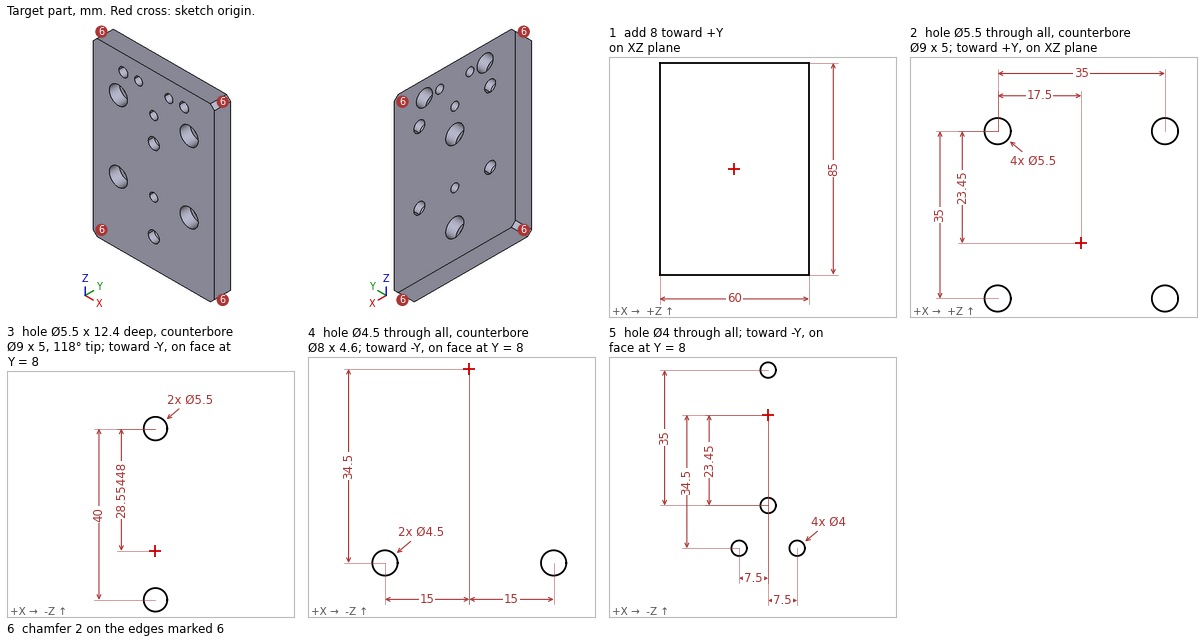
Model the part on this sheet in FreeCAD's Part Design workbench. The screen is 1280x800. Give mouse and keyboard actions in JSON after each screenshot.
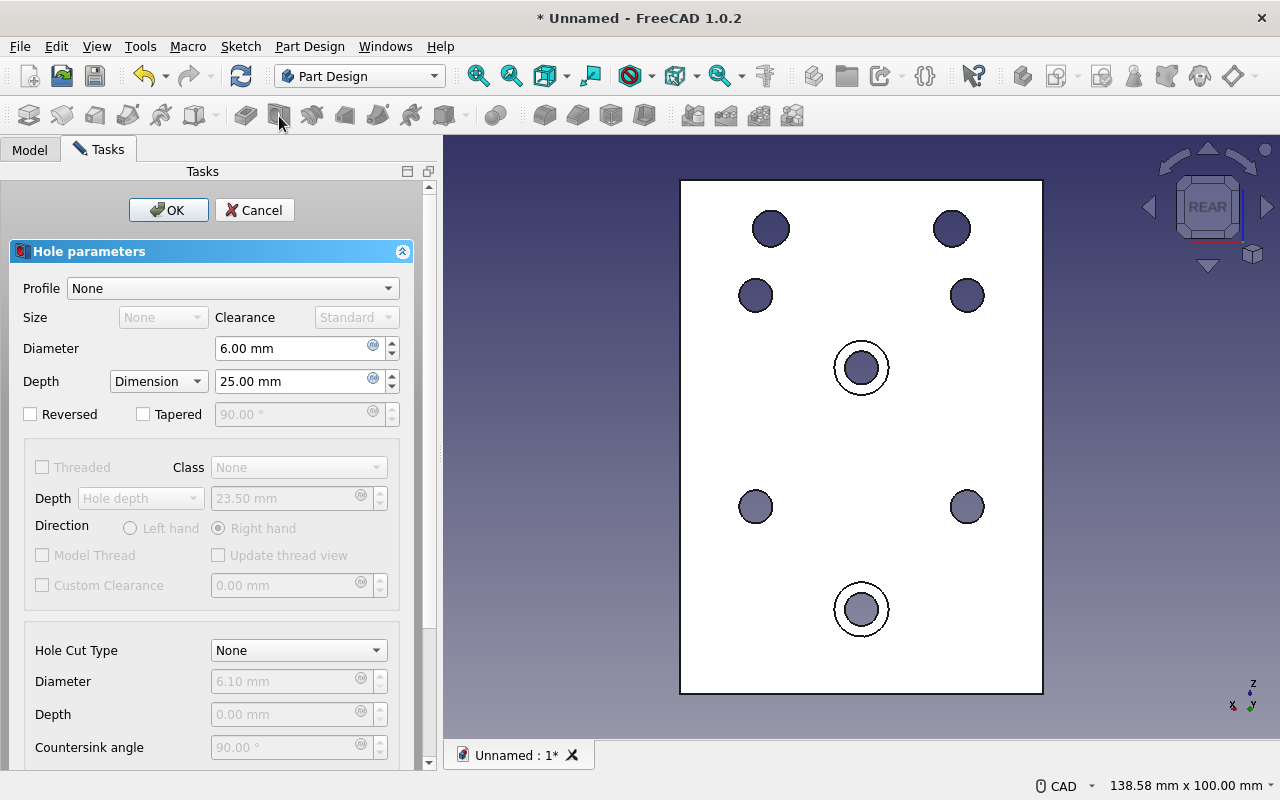
{"action": "triple_click", "coordinate": [300, 348]}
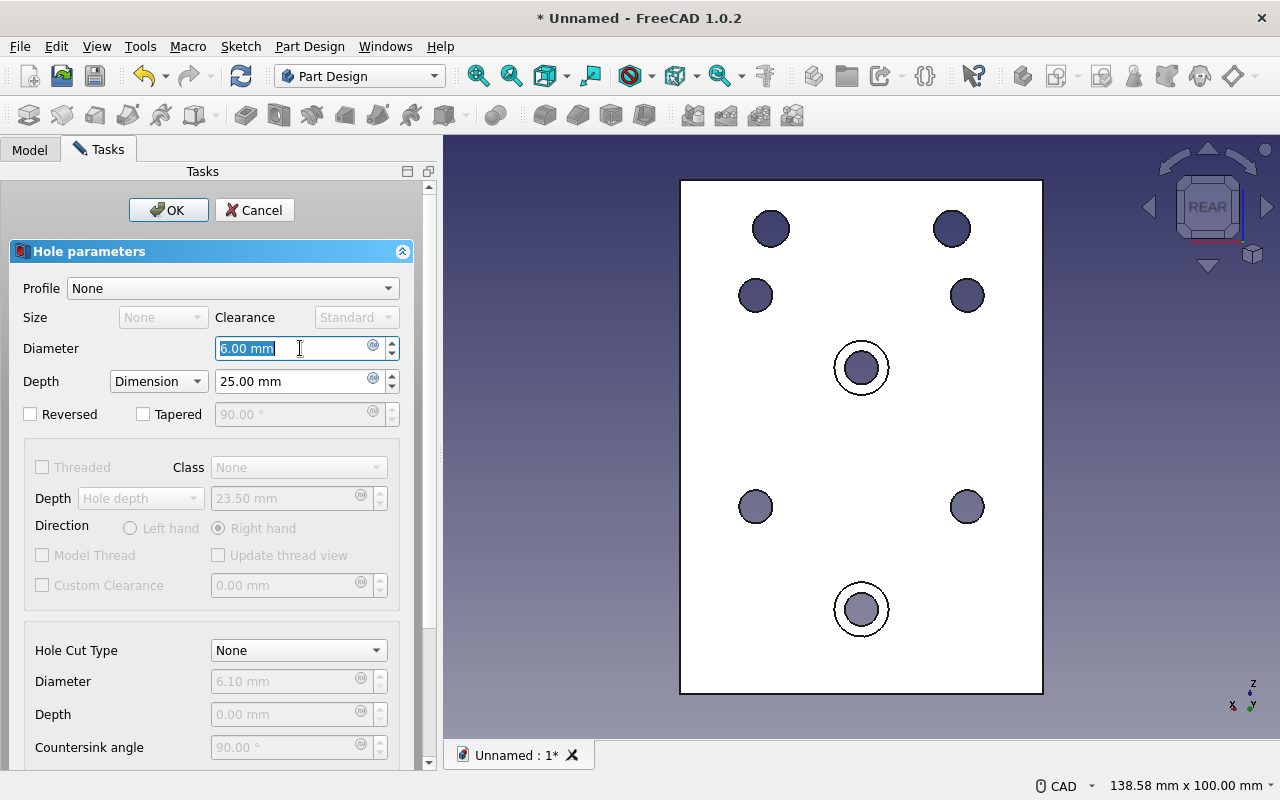
{"action": "type", "text": "4.5"}
{"action": "key", "text": "Tab"}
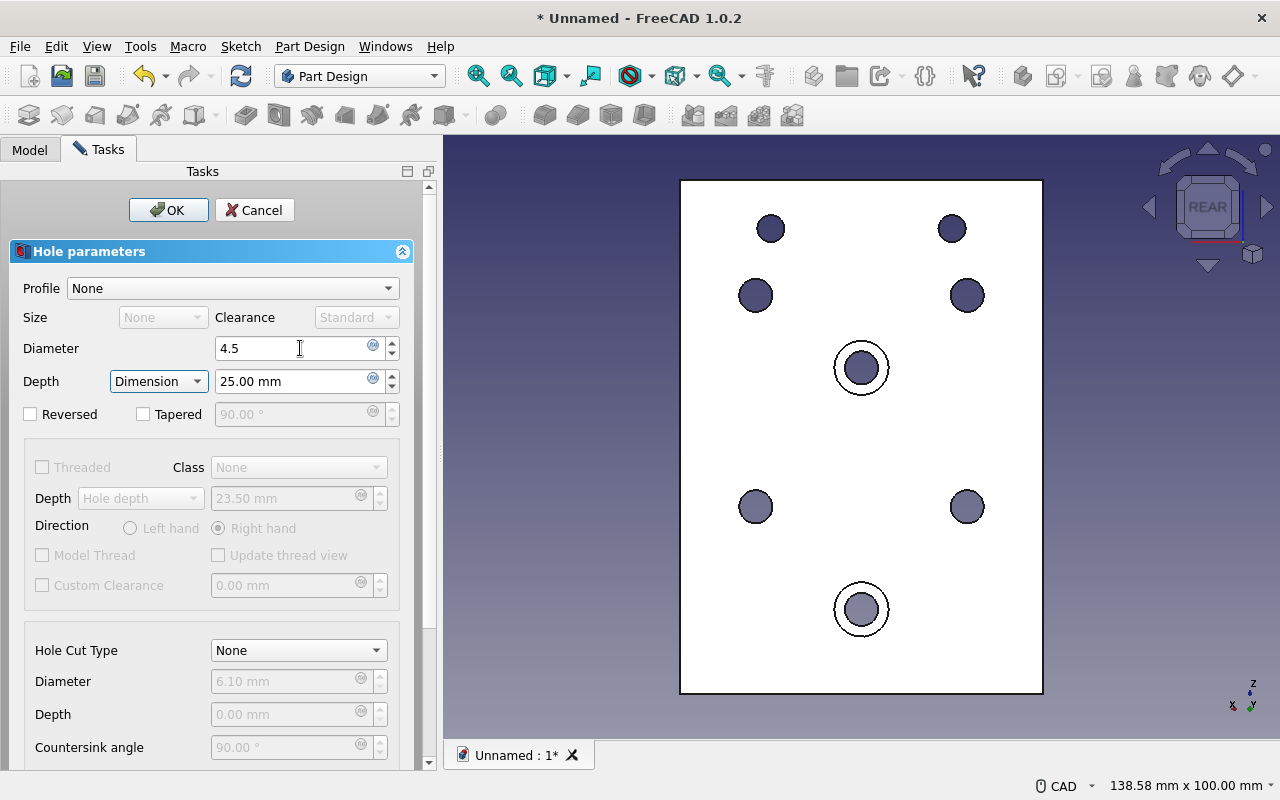
{"action": "left_click", "coordinate": [160, 382]}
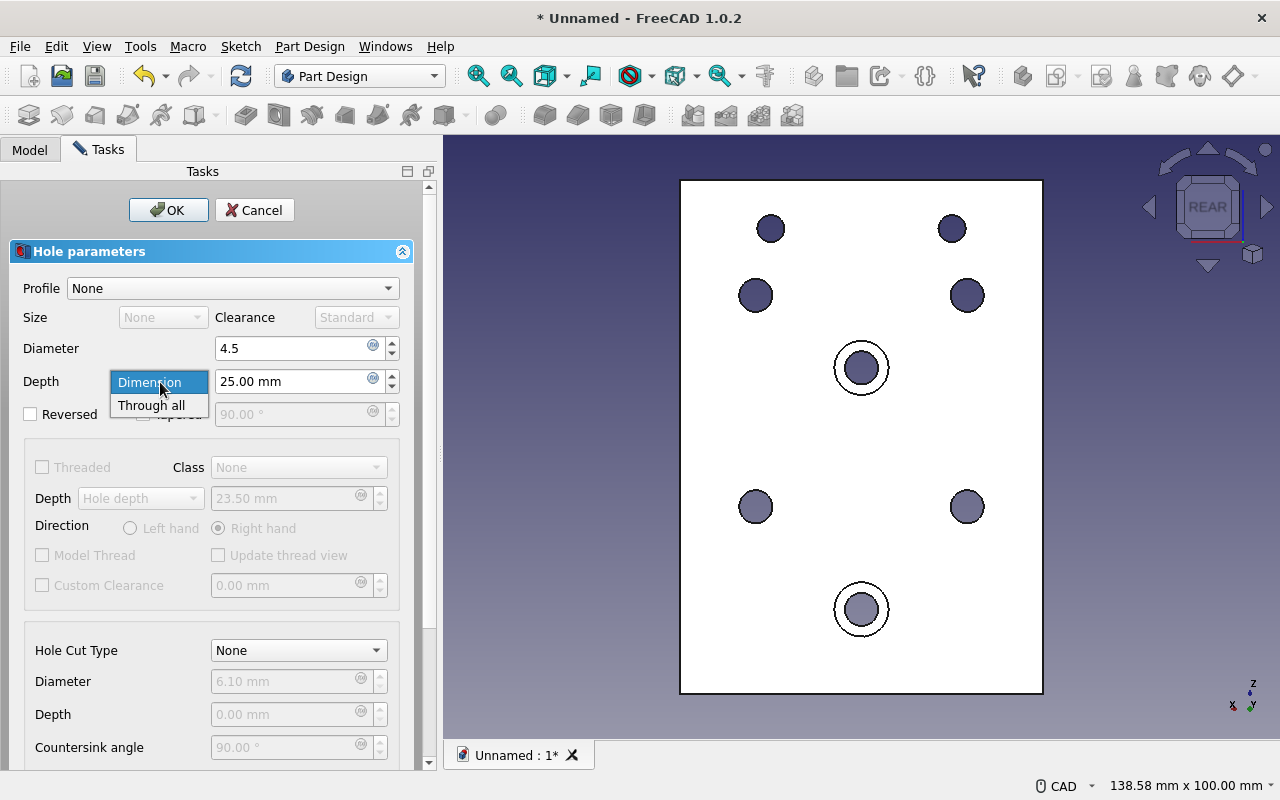
{"action": "left_click", "coordinate": [158, 406]}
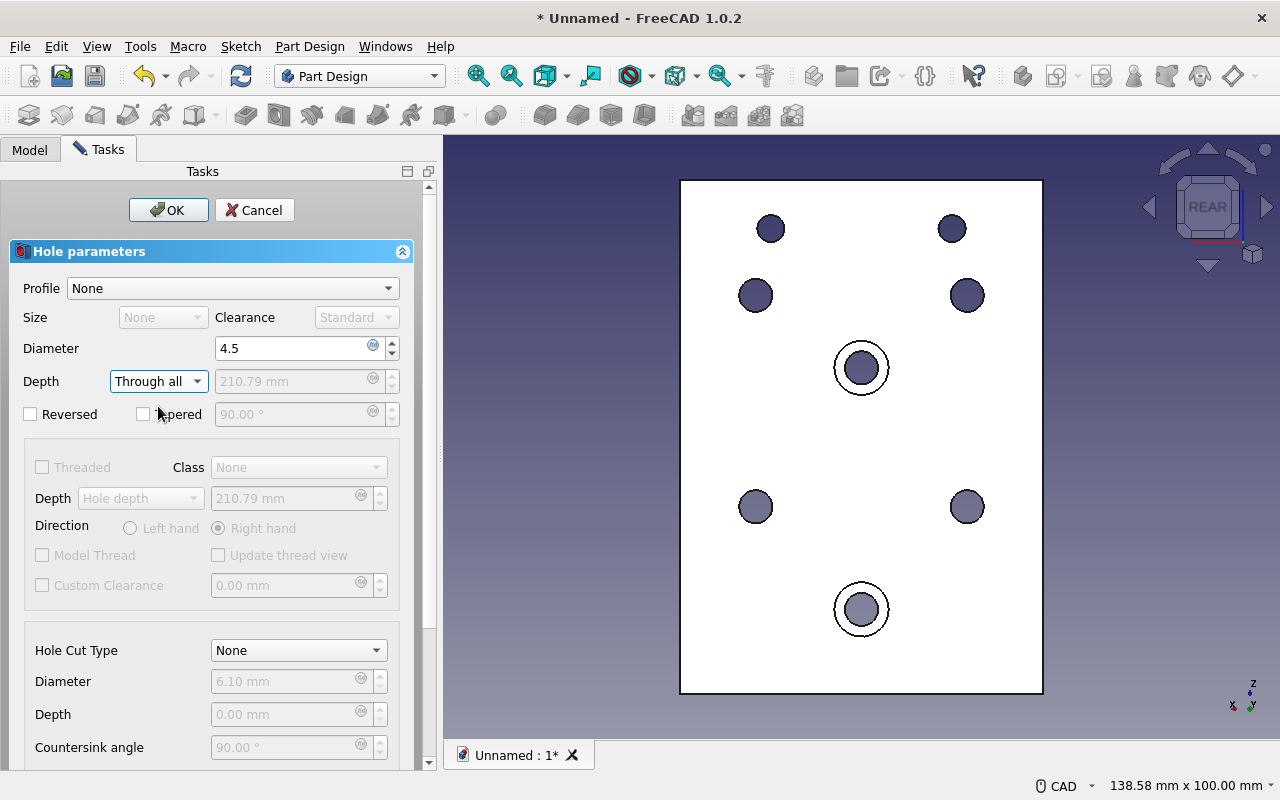
{"action": "left_click", "coordinate": [300, 650]}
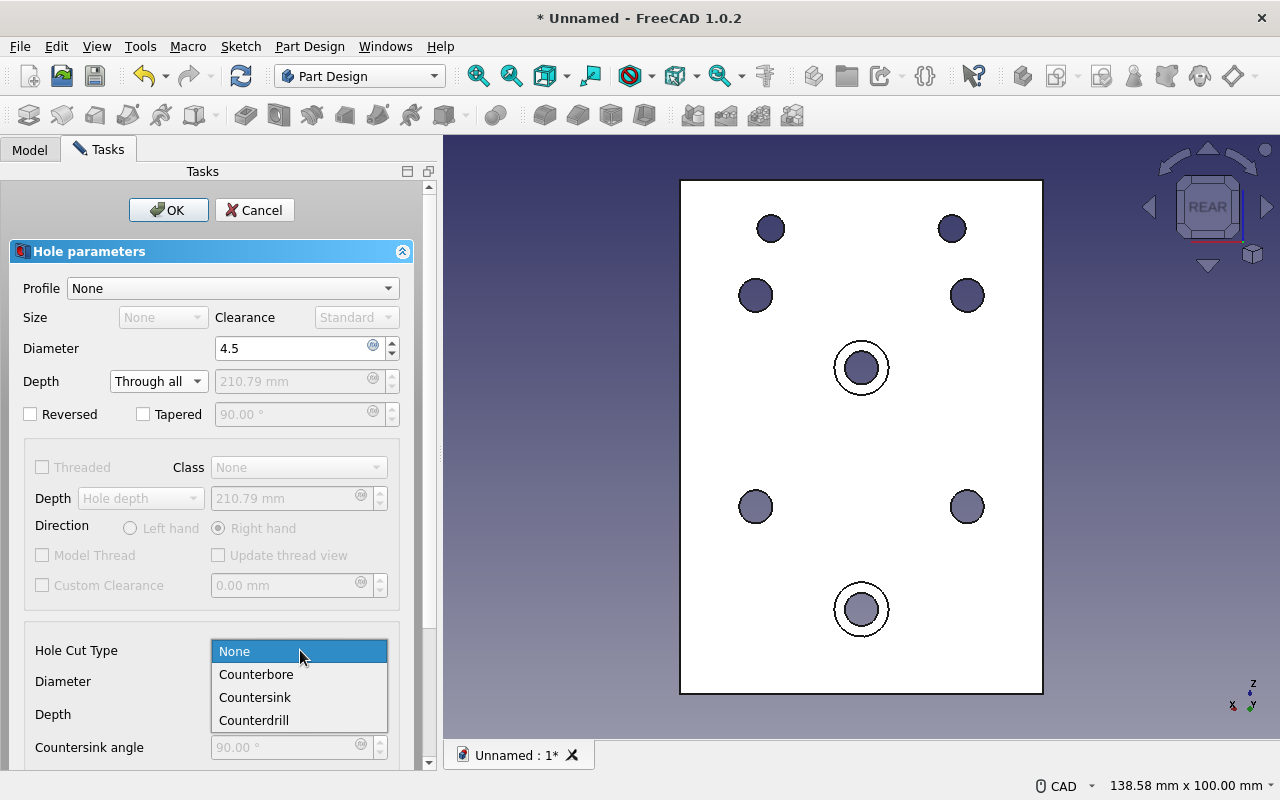
{"action": "left_click", "coordinate": [298, 674]}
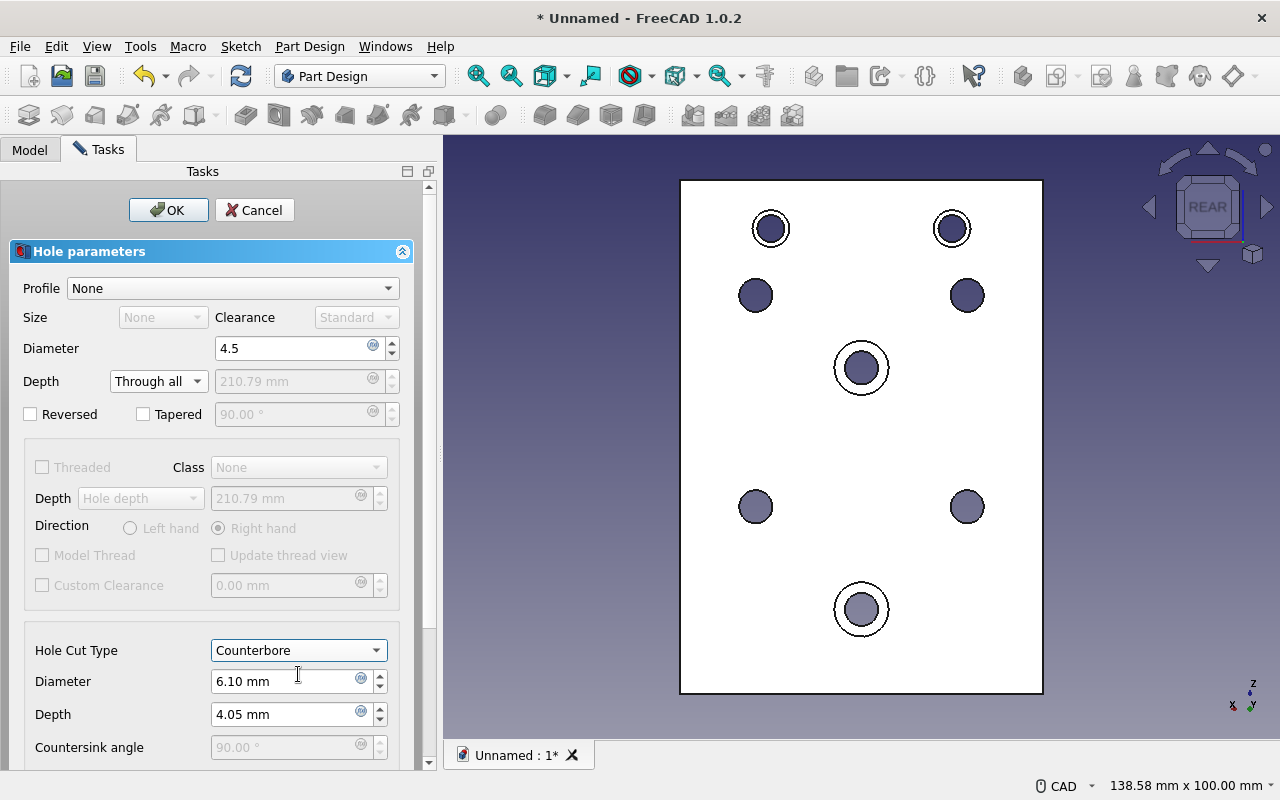
{"action": "triple_click", "coordinate": [292, 682]}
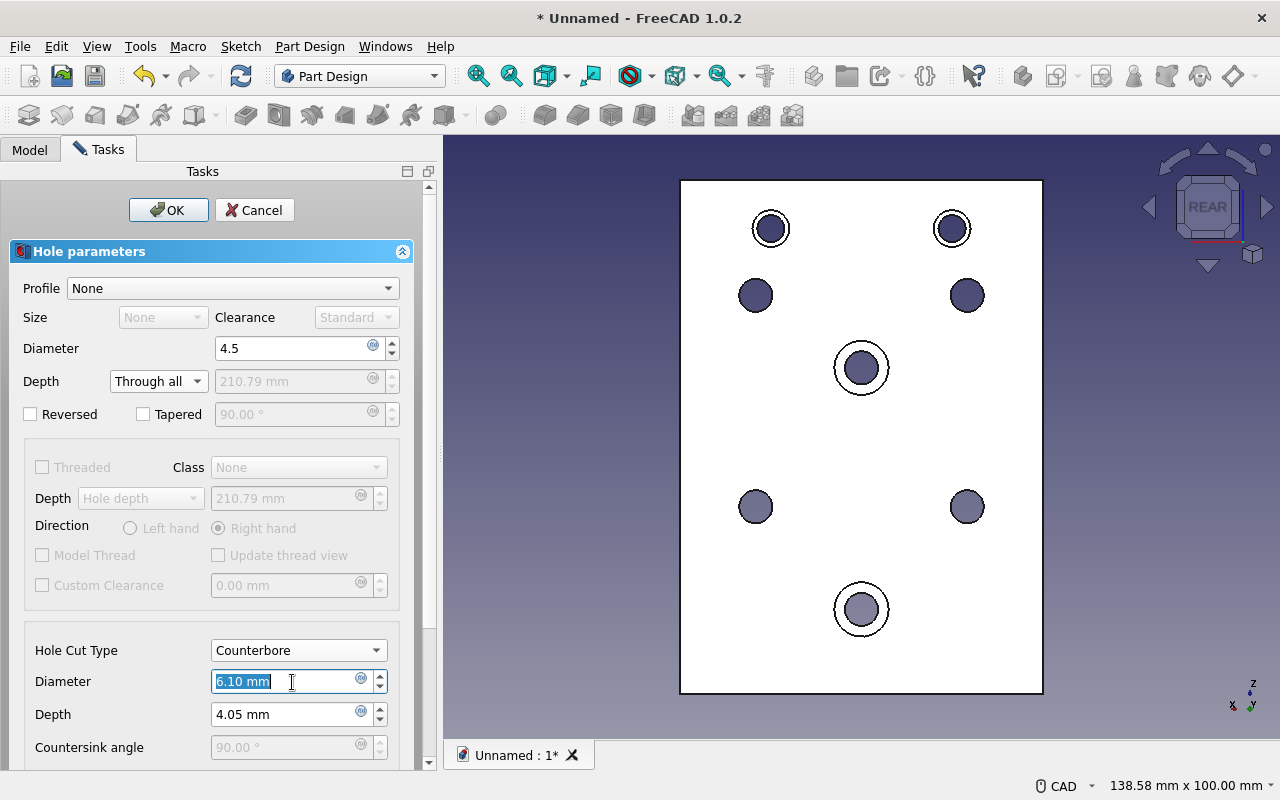
{"action": "type", "text": "8"}
{"action": "key", "text": "Tab"}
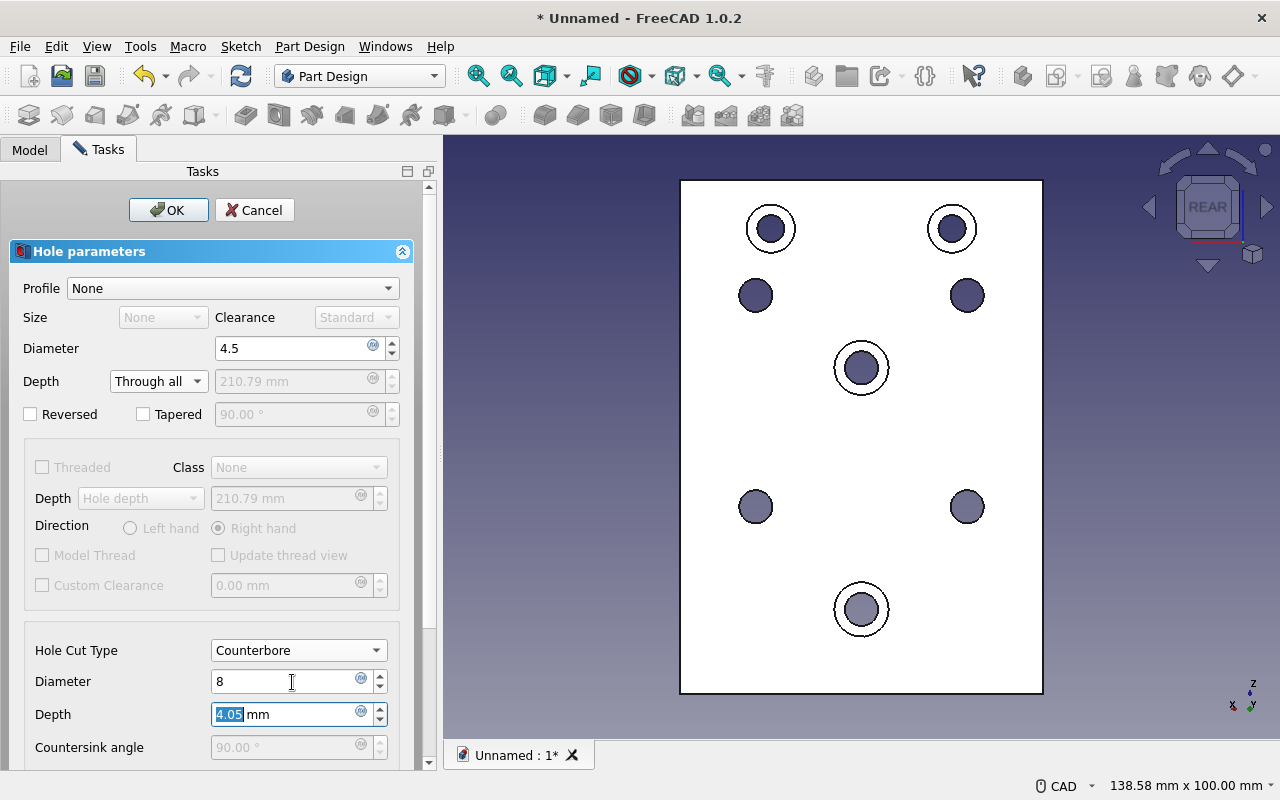
{"action": "type", "text": "4.6"}
{"action": "key", "text": "Tab"}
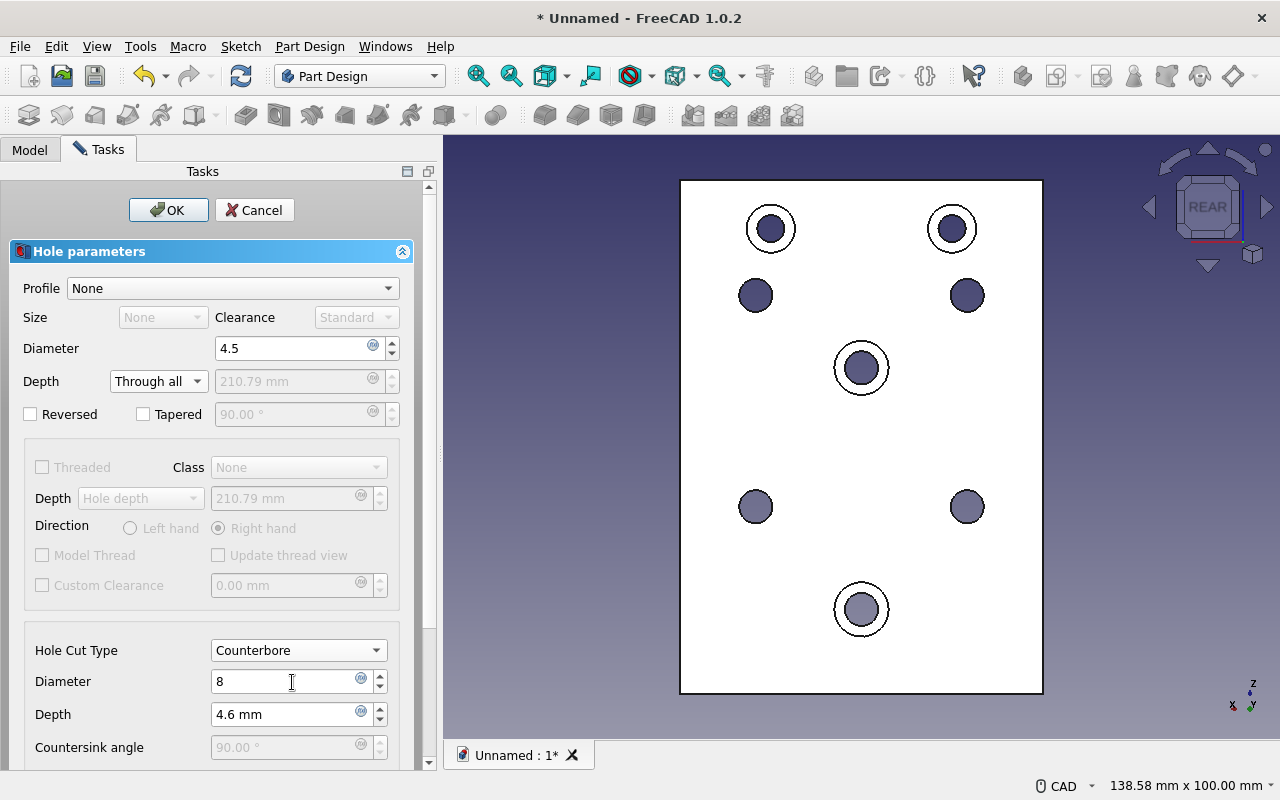
{"action": "left_click", "coordinate": [169, 210]}